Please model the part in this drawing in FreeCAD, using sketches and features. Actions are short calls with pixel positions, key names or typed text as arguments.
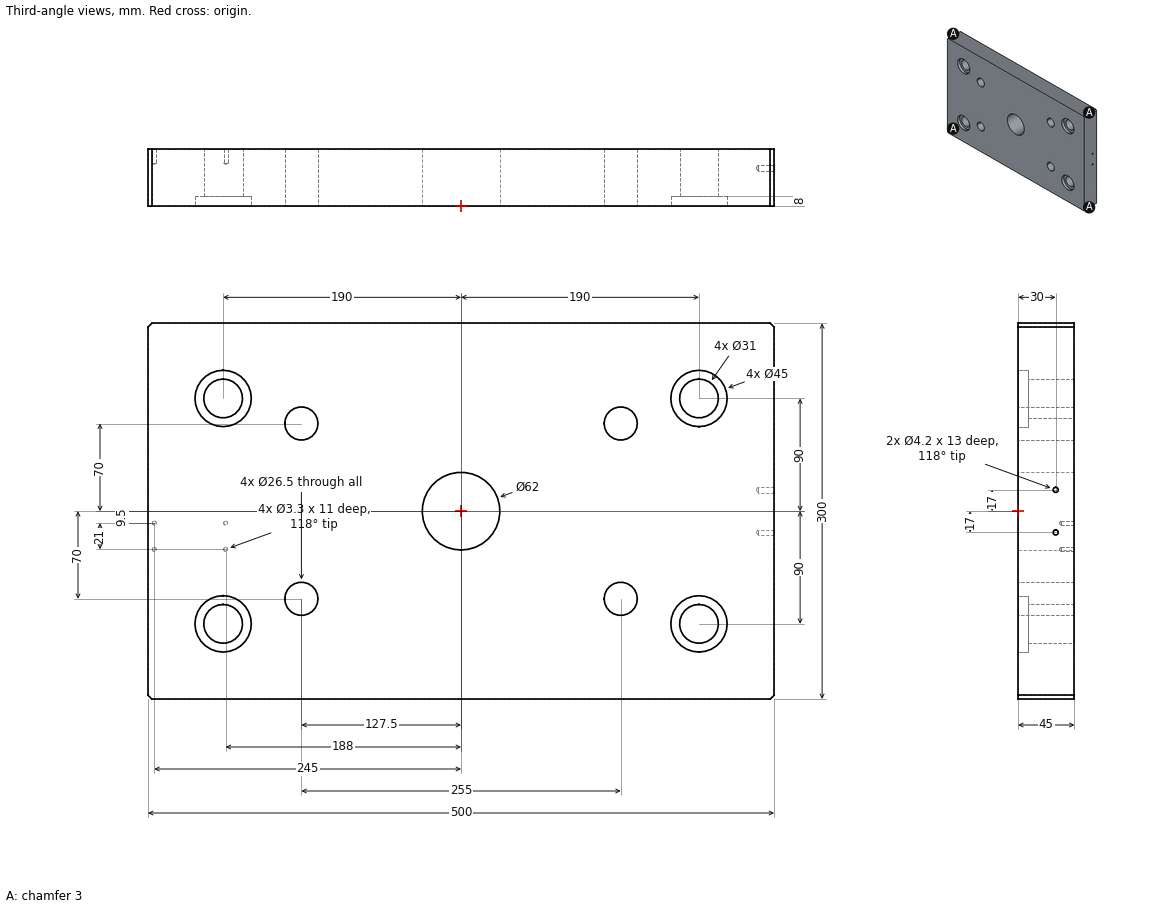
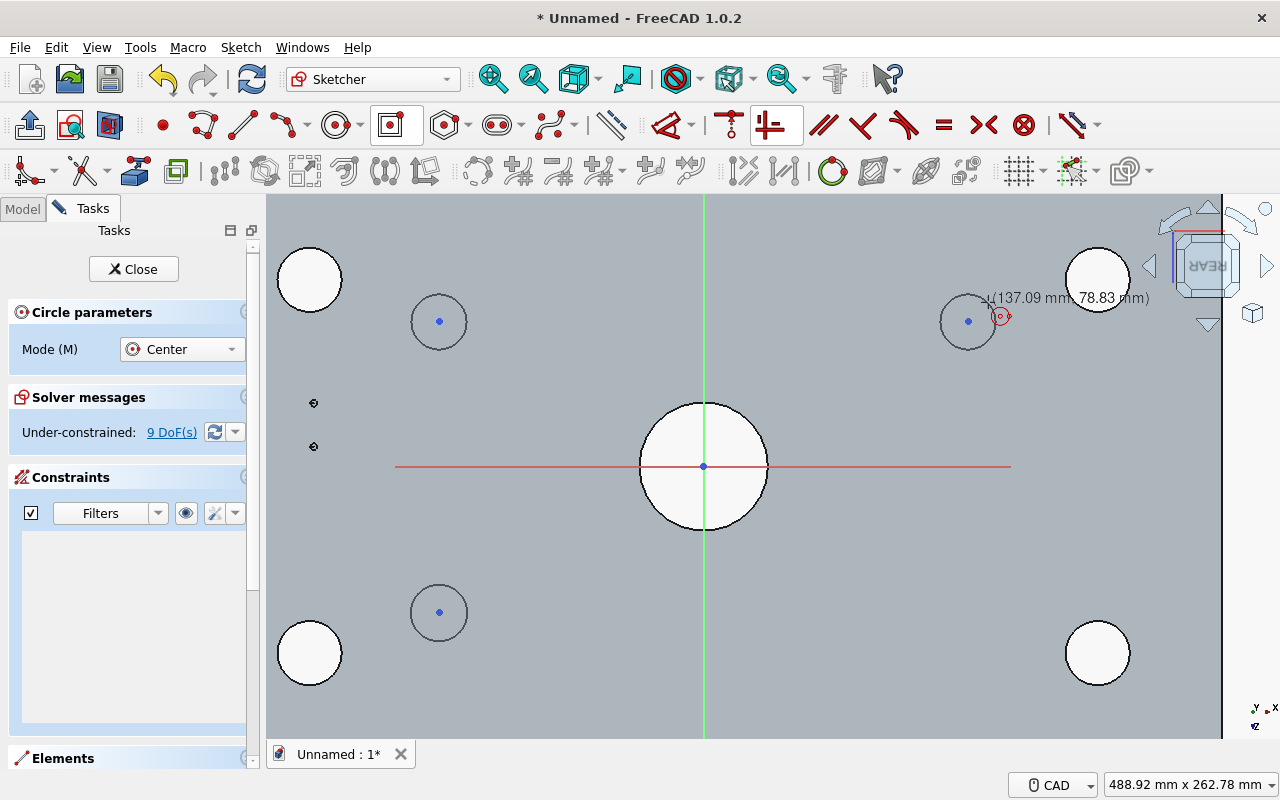
click(968, 612)
click(988, 592)
key(Escape)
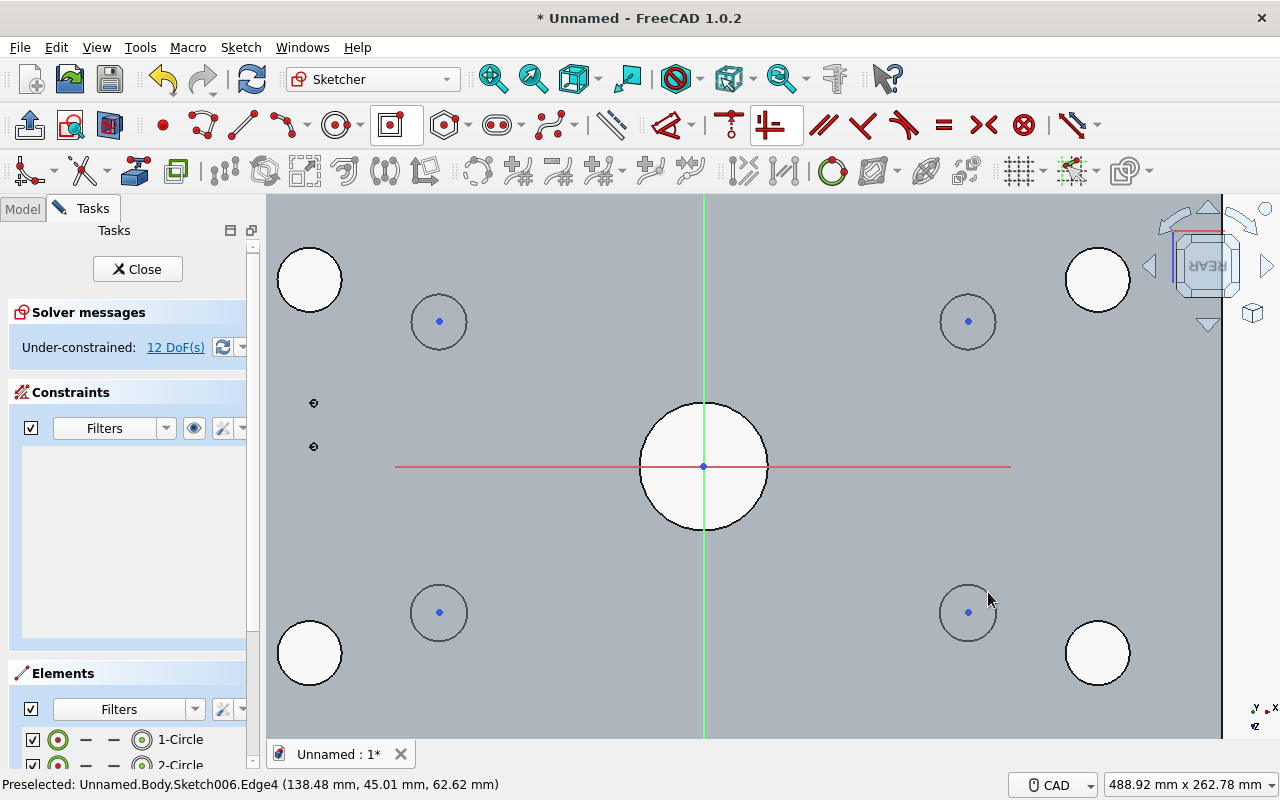
click(458, 302)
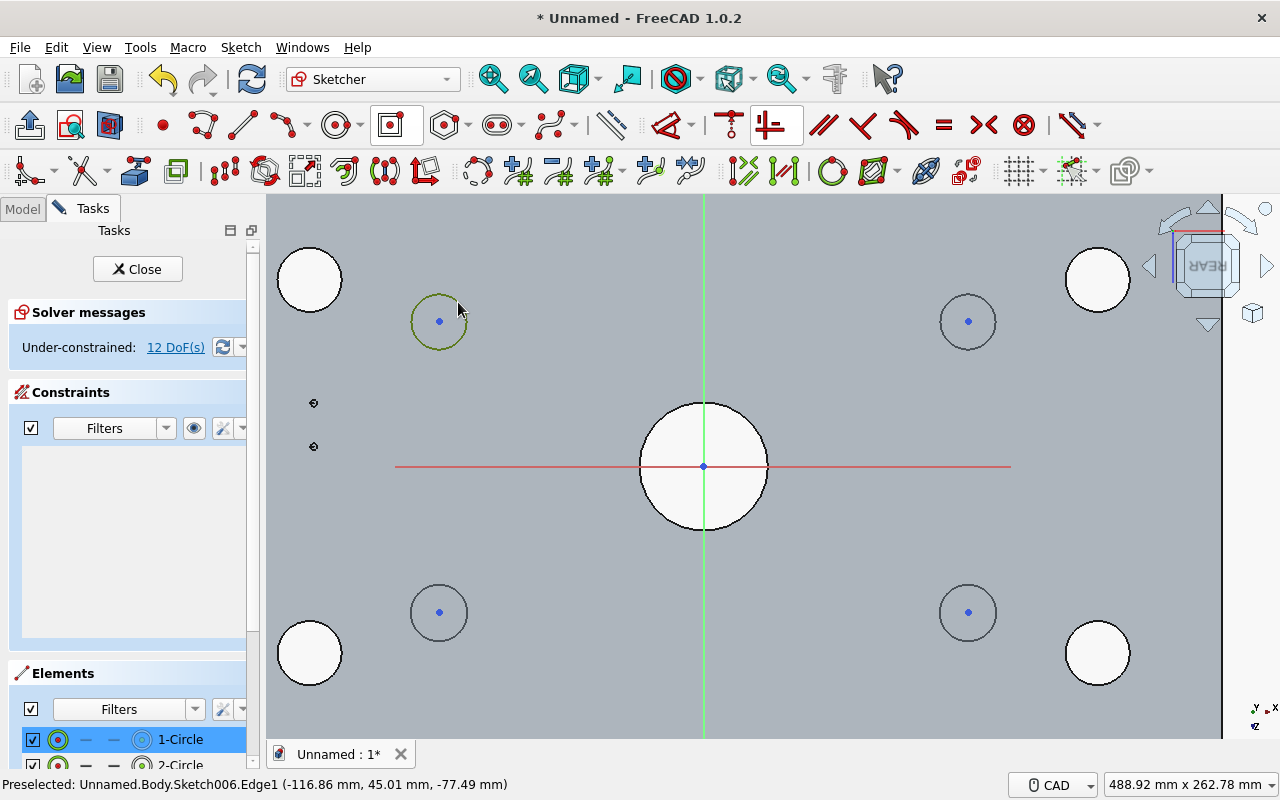
click(459, 593)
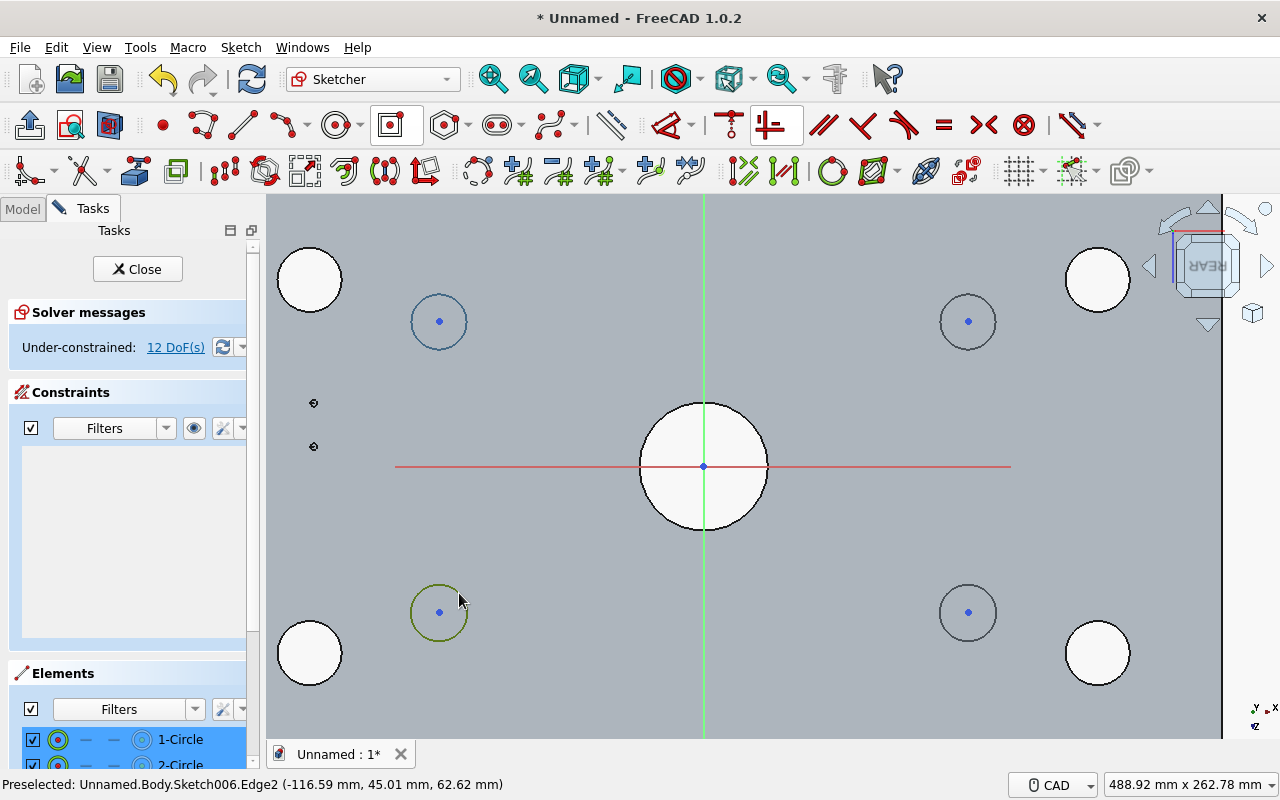
click(987, 302)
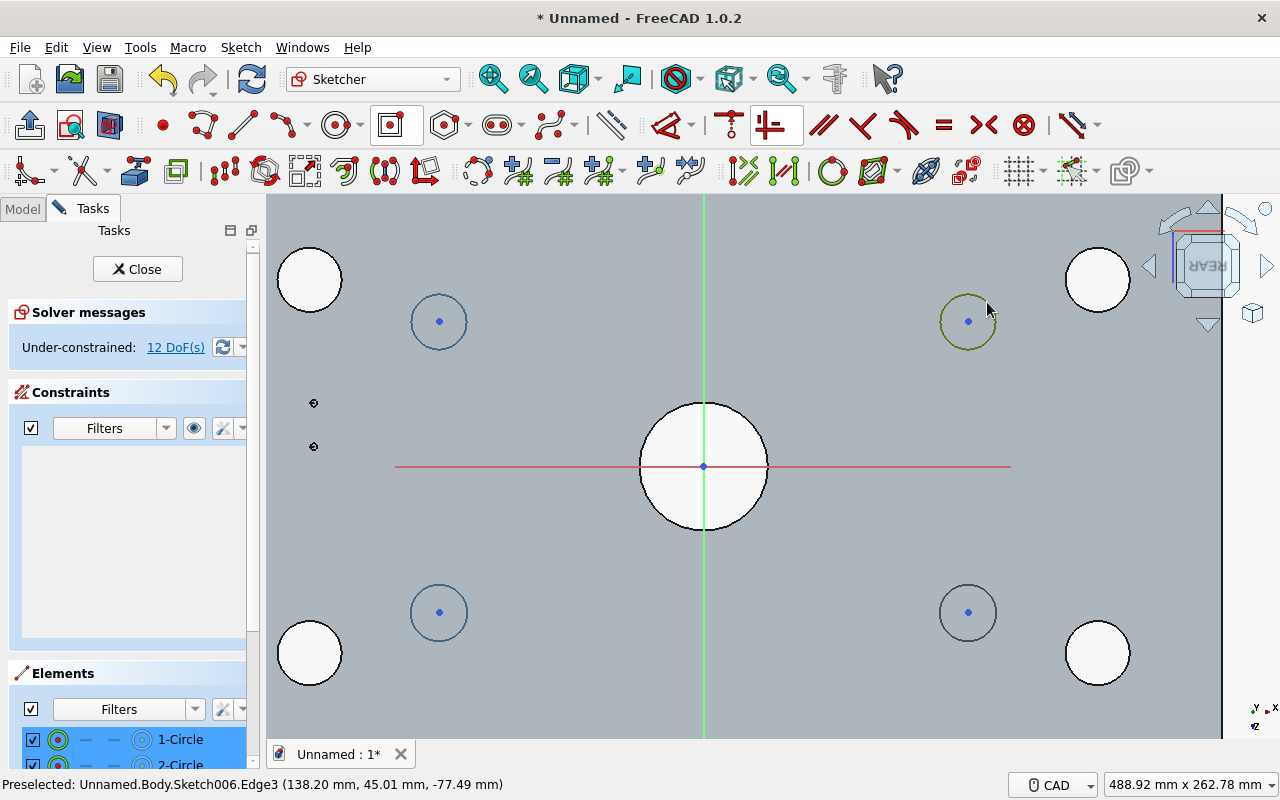
click(988, 593)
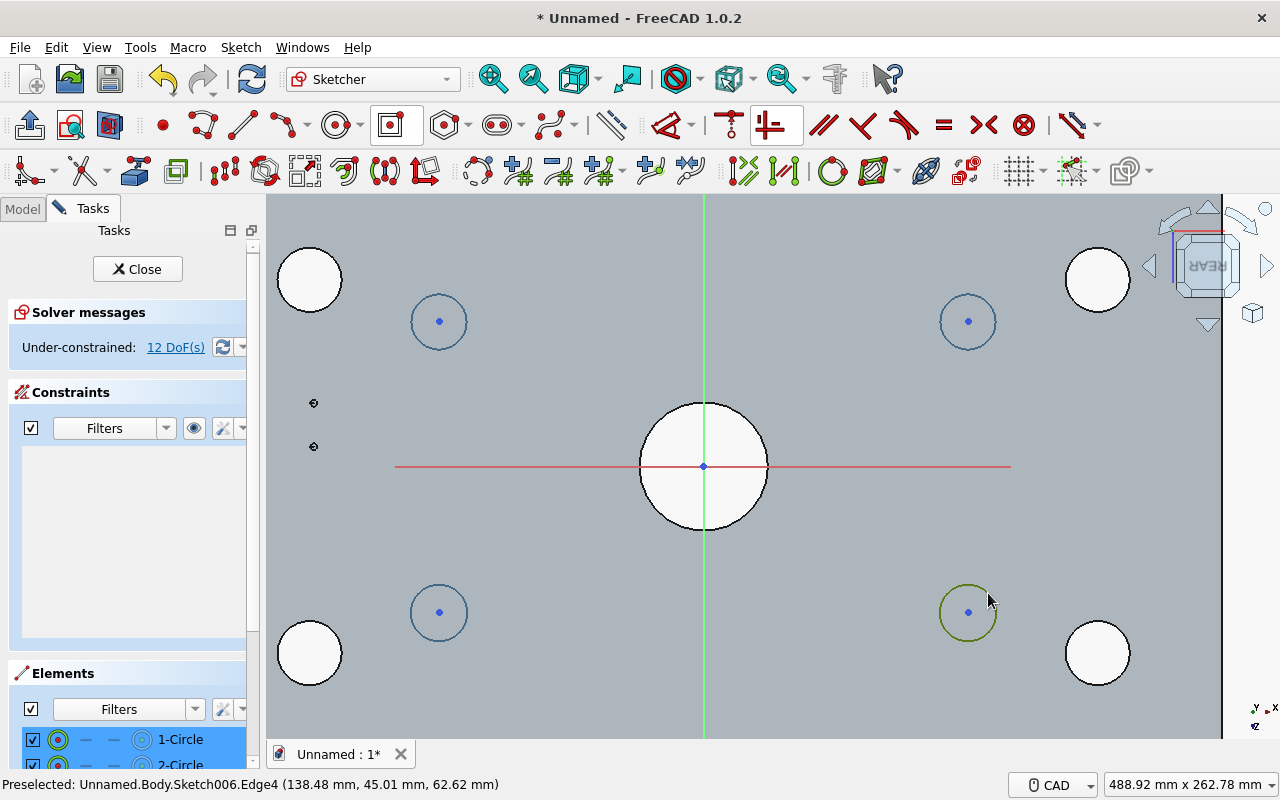
click(944, 126)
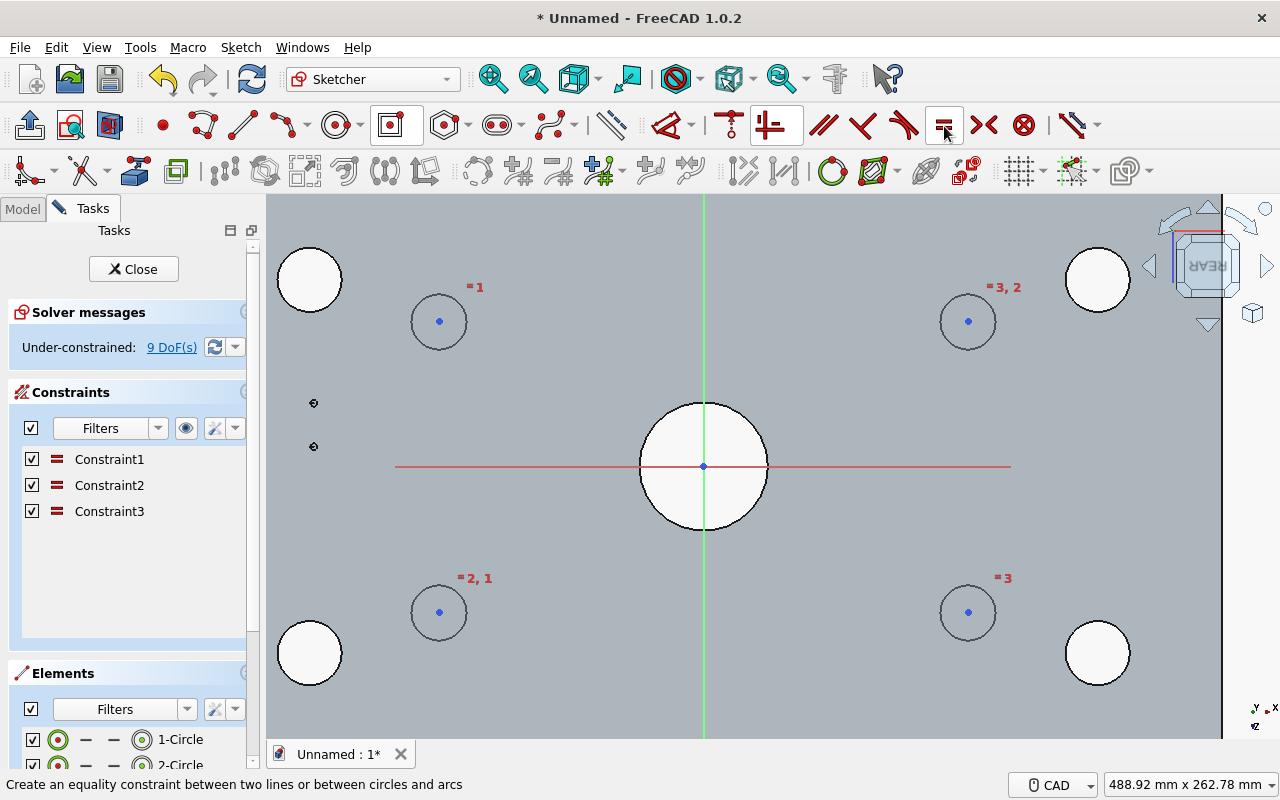
click(439, 322)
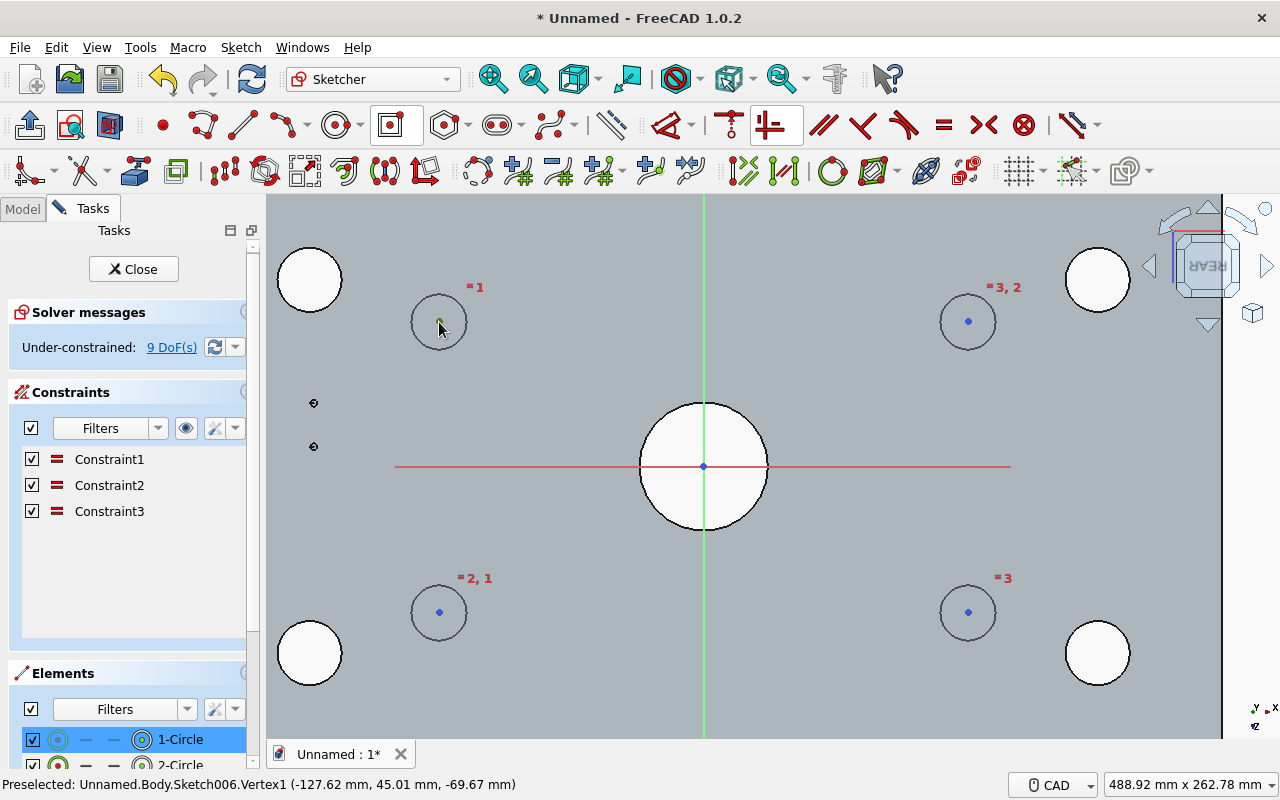
click(439, 613)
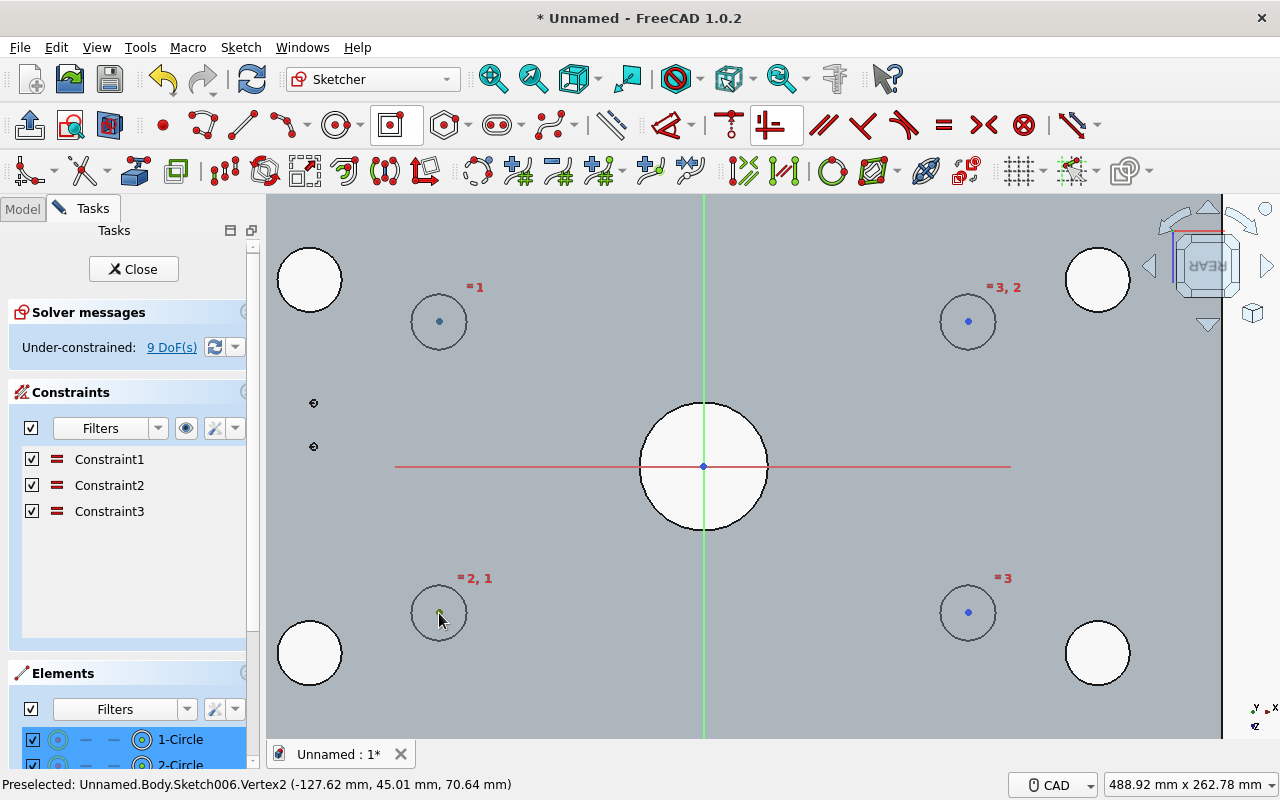
click(798, 126)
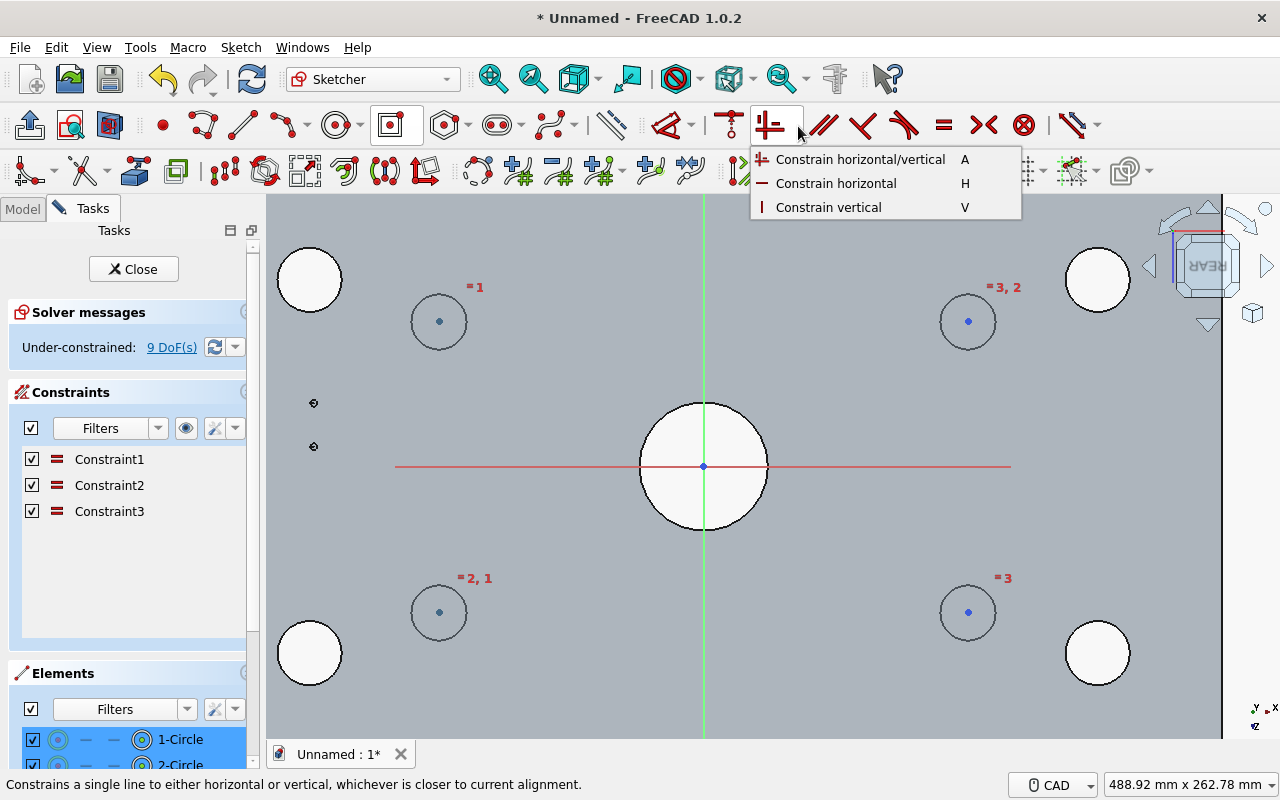
click(886, 207)